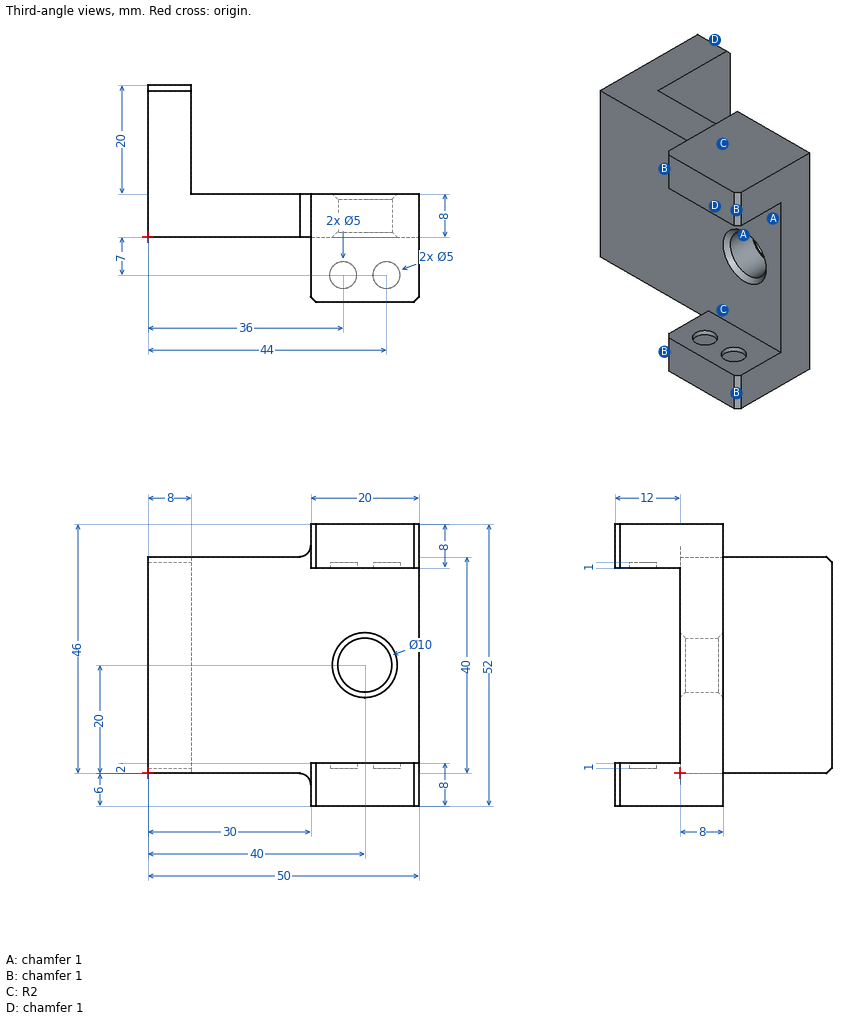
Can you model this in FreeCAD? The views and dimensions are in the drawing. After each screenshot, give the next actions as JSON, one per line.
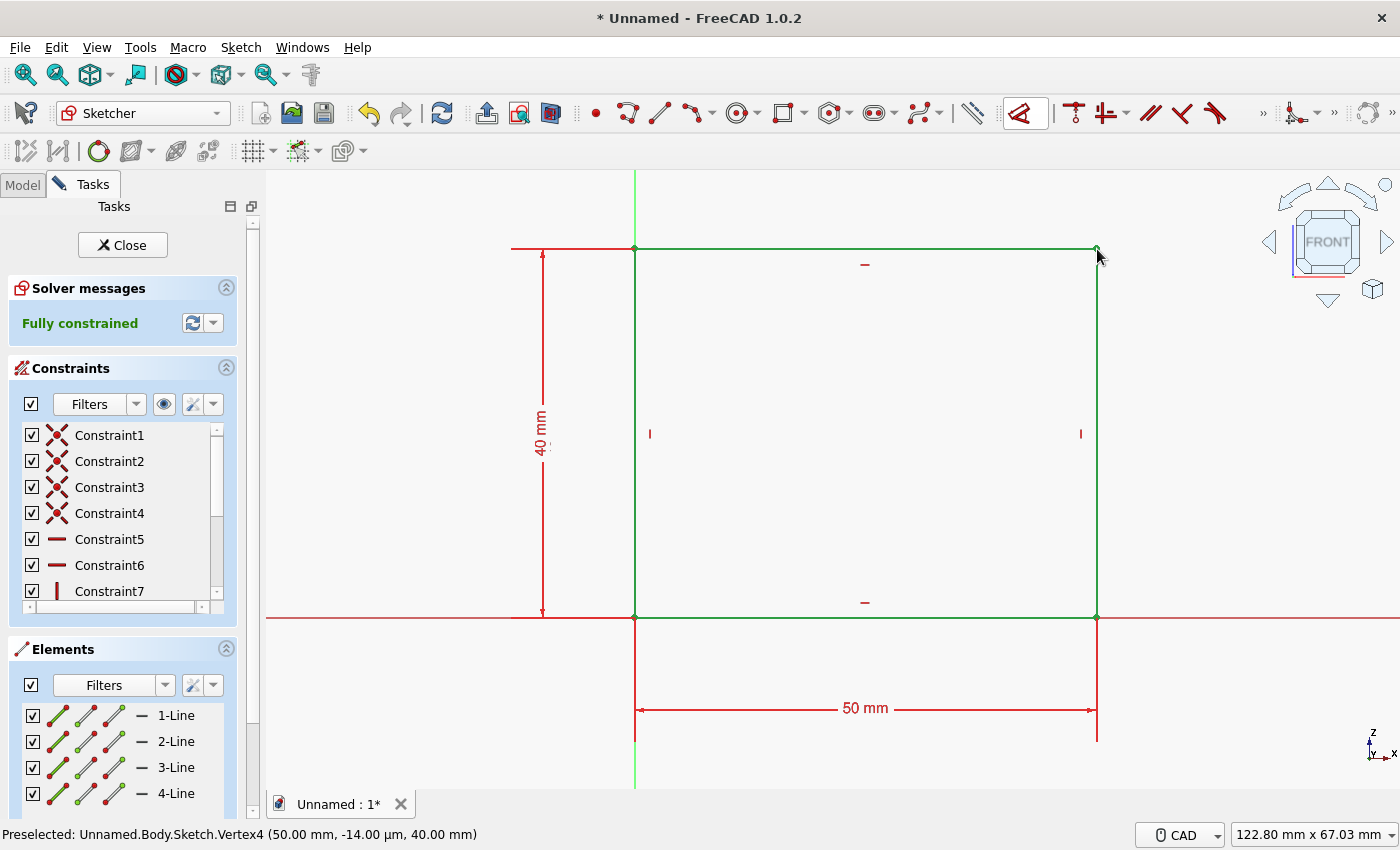
{"action": "left_click", "coordinate": [123, 245]}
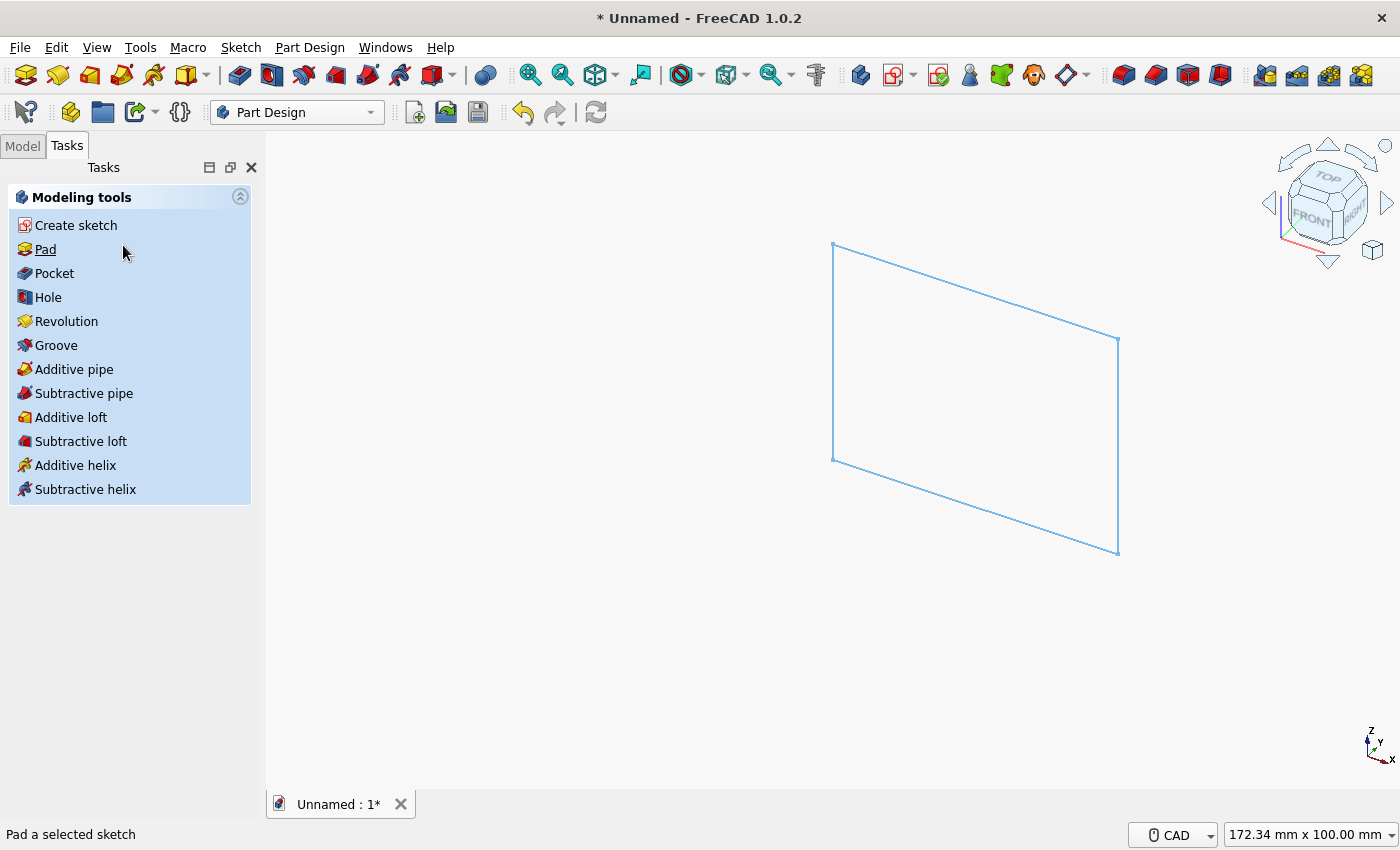
{"action": "left_click", "coordinate": [26, 76]}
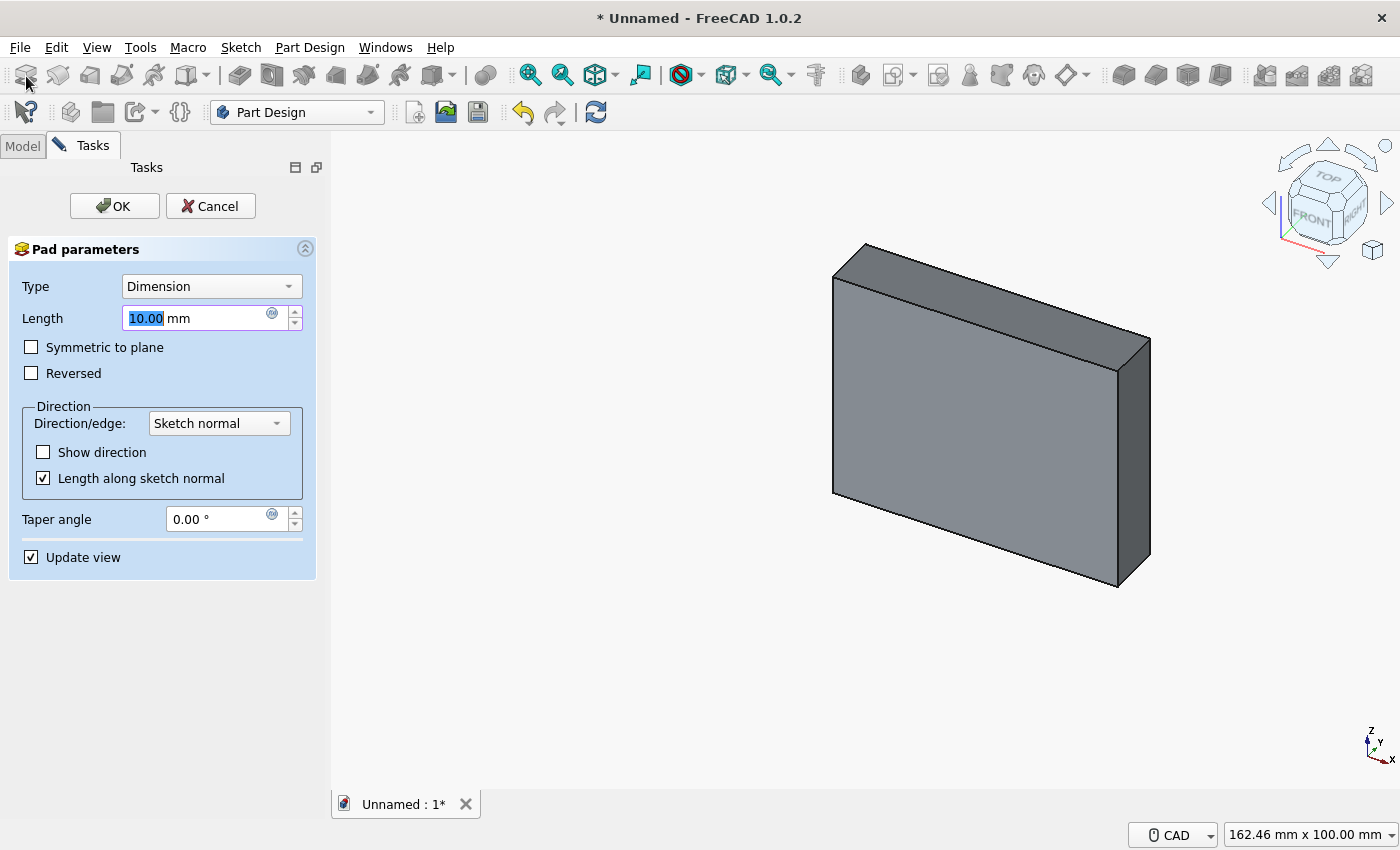
{"action": "type", "text": "8"}
{"action": "key", "text": "Tab"}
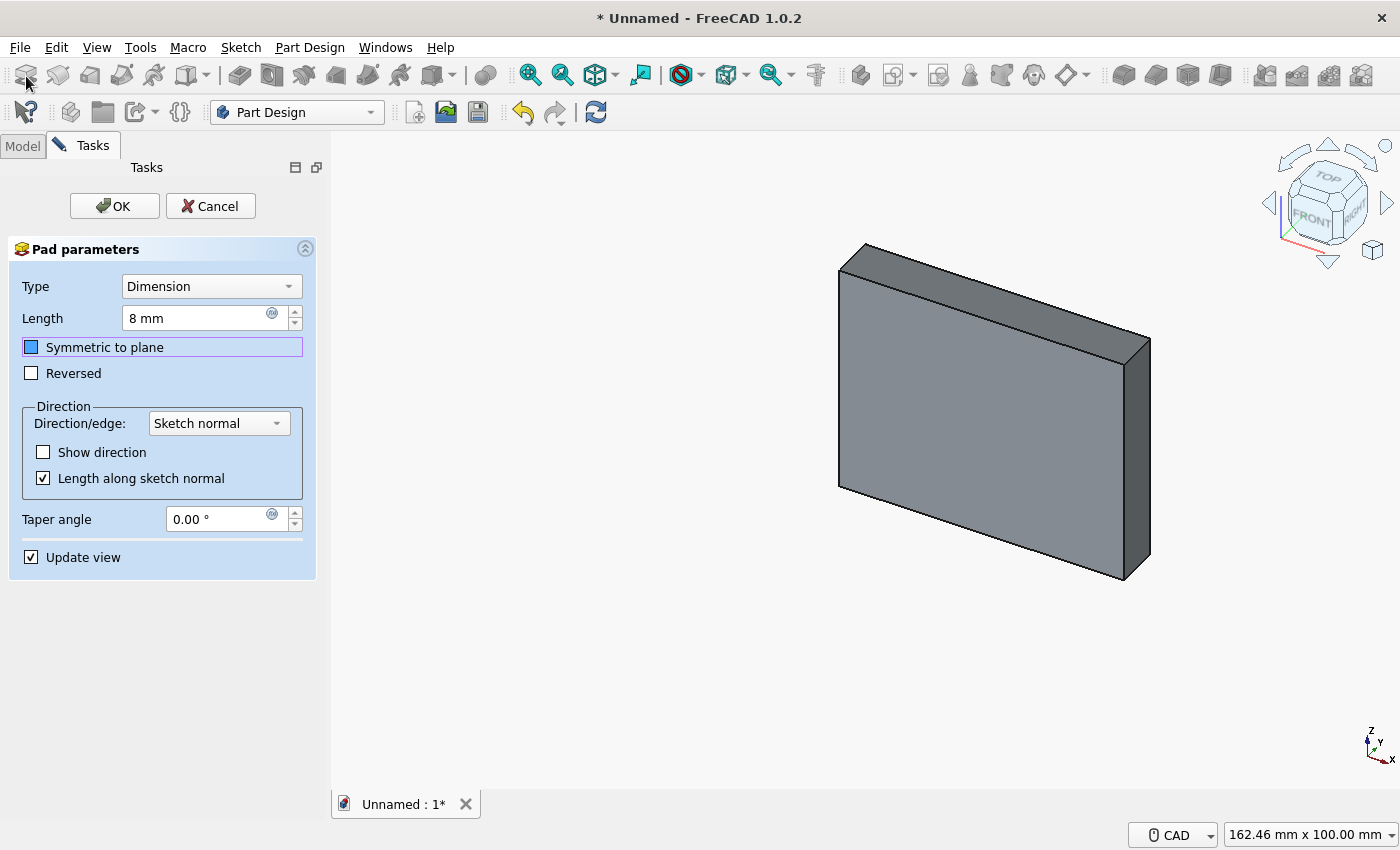
{"action": "left_click", "coordinate": [30, 373]}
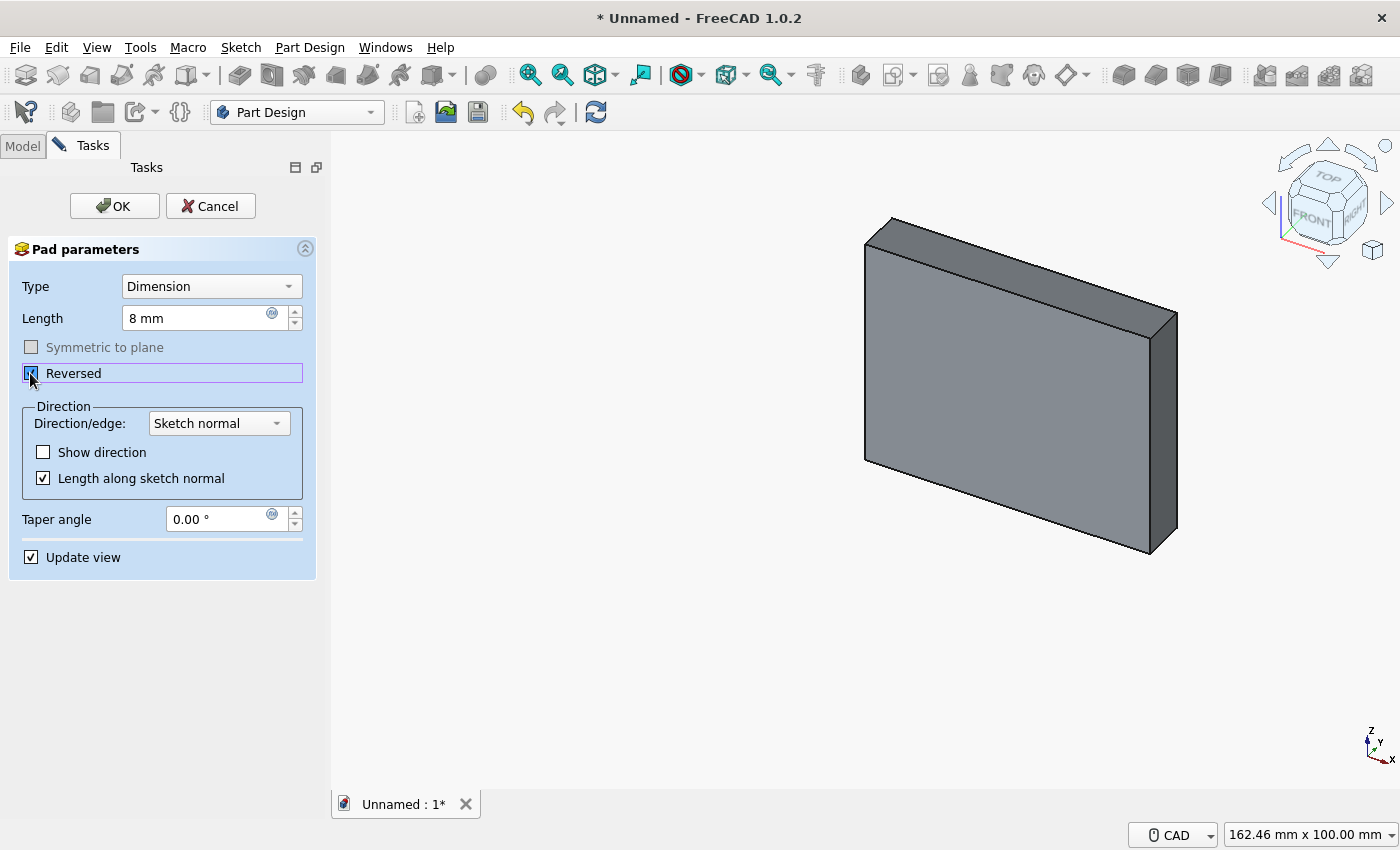
{"action": "left_click", "coordinate": [115, 206]}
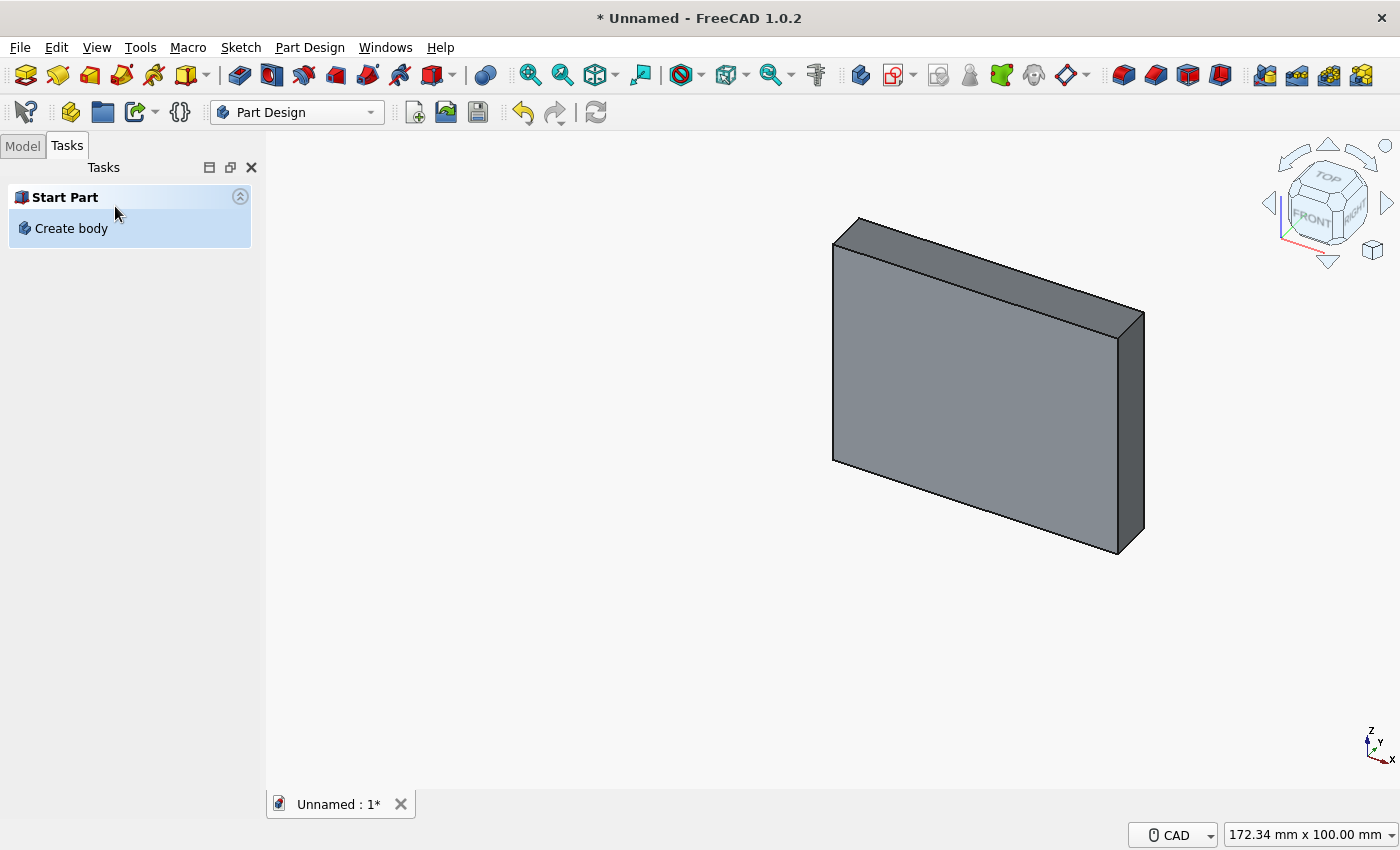
{"action": "key", "text": "4"}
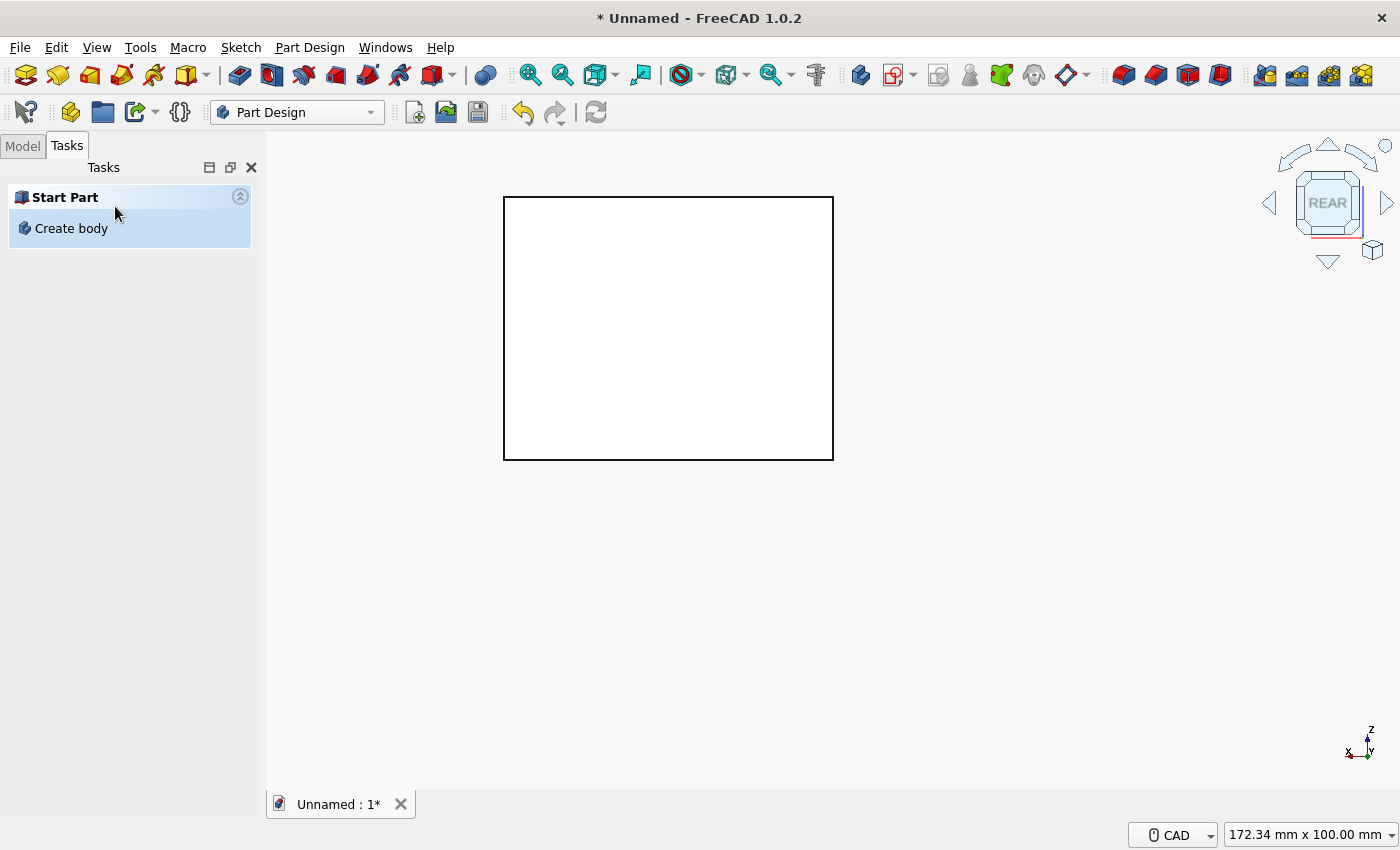
{"action": "left_click", "coordinate": [532, 76]}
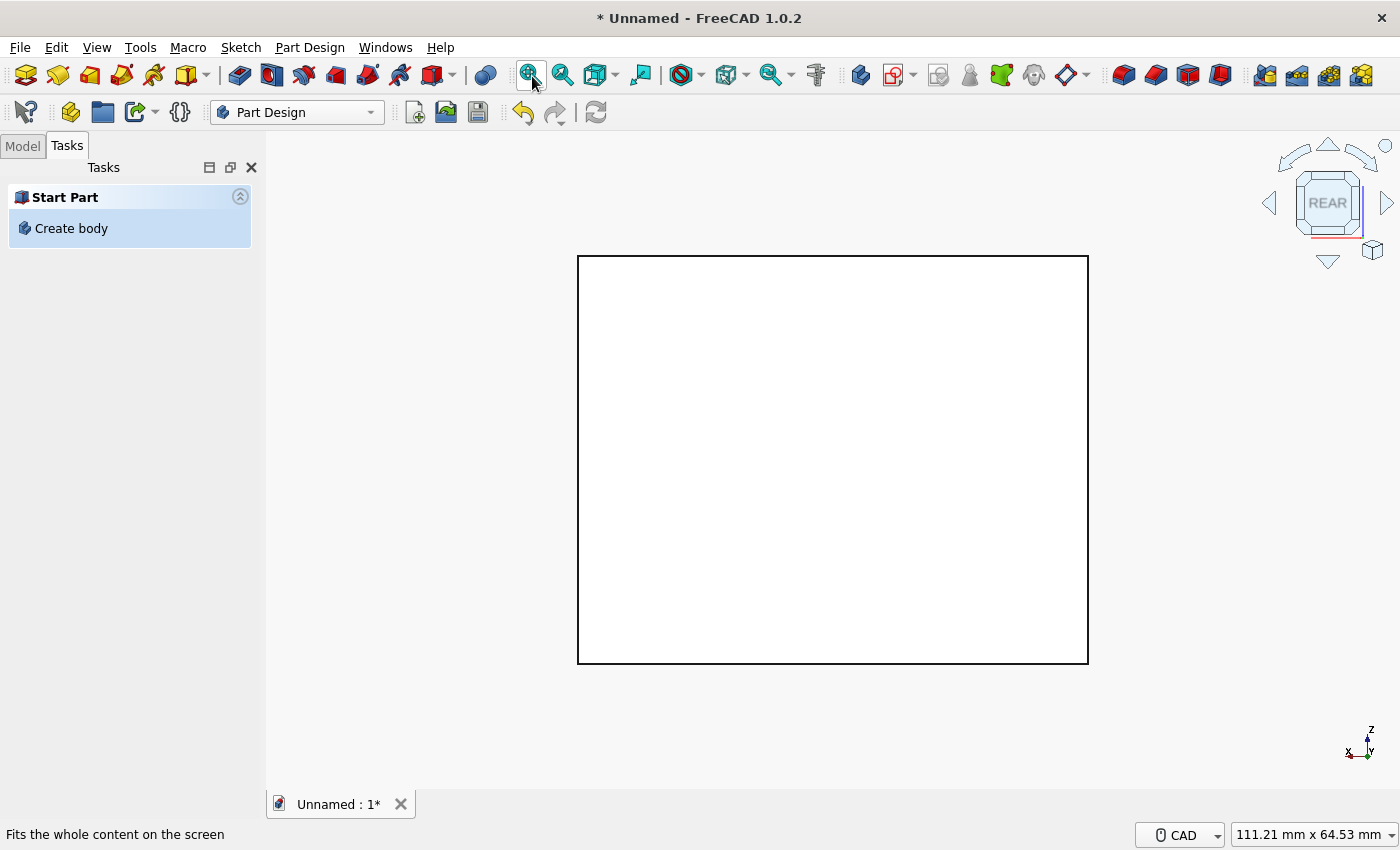
{"action": "left_click", "coordinate": [833, 459]}